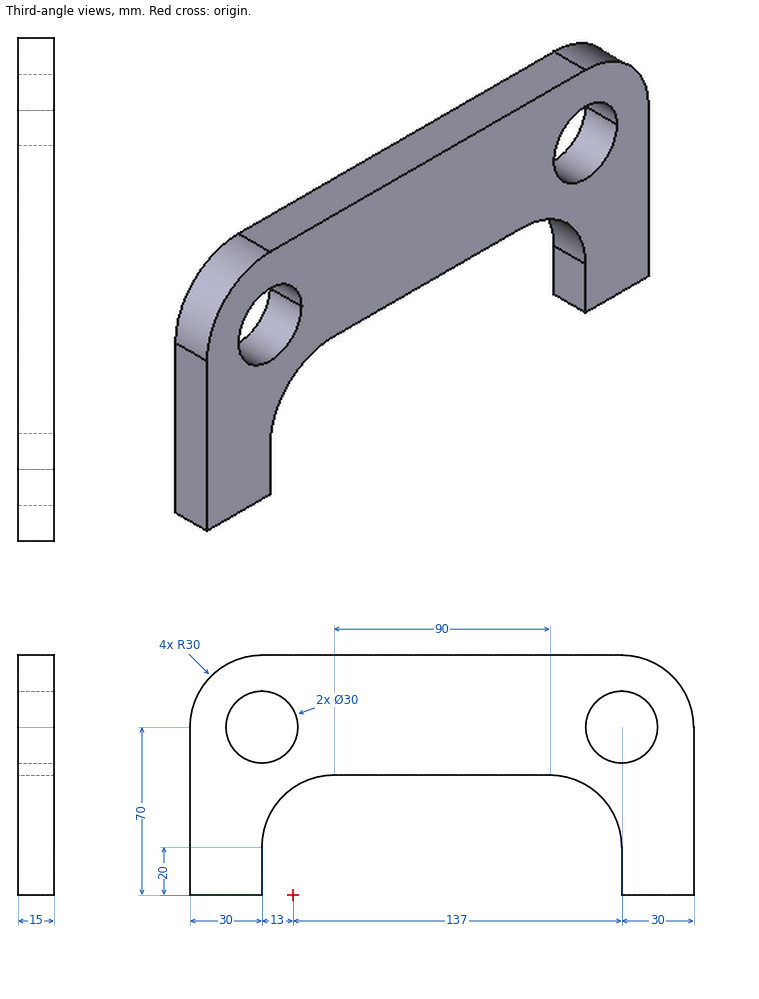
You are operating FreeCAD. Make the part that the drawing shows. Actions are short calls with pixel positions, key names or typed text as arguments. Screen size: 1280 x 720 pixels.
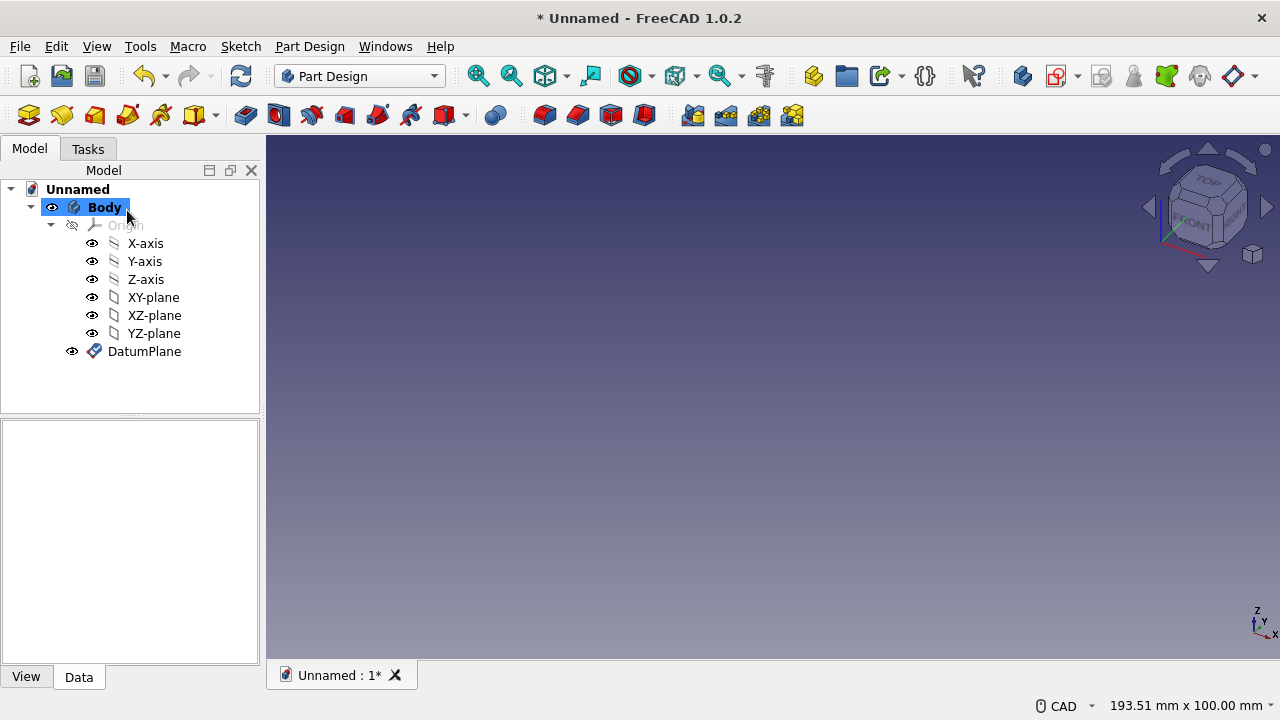
click(117, 351)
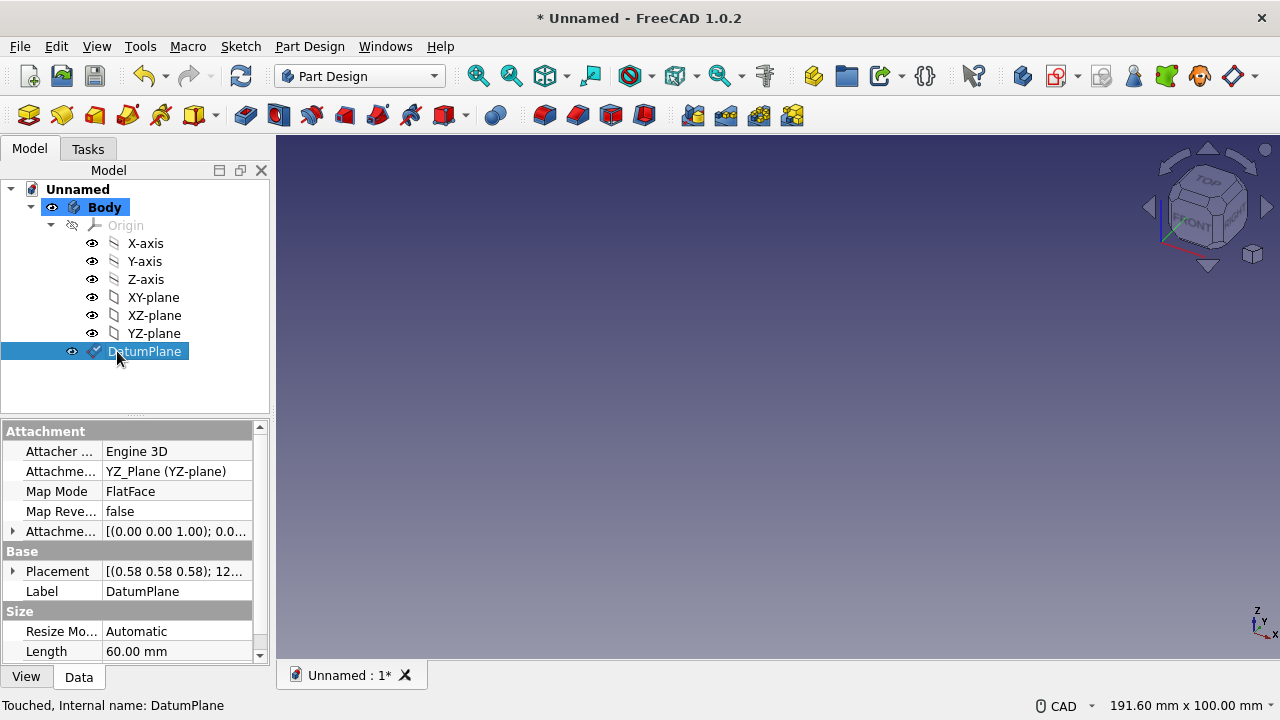
click(1056, 76)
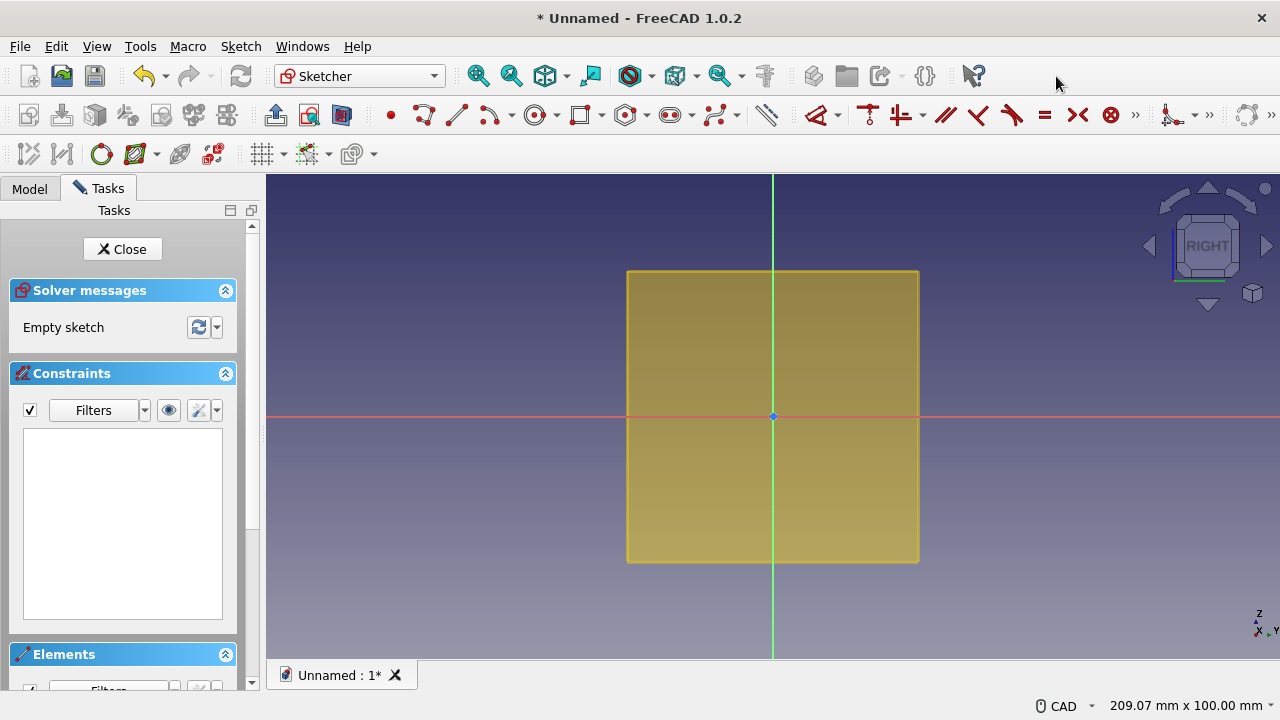
scroll(294, 631, down, 3)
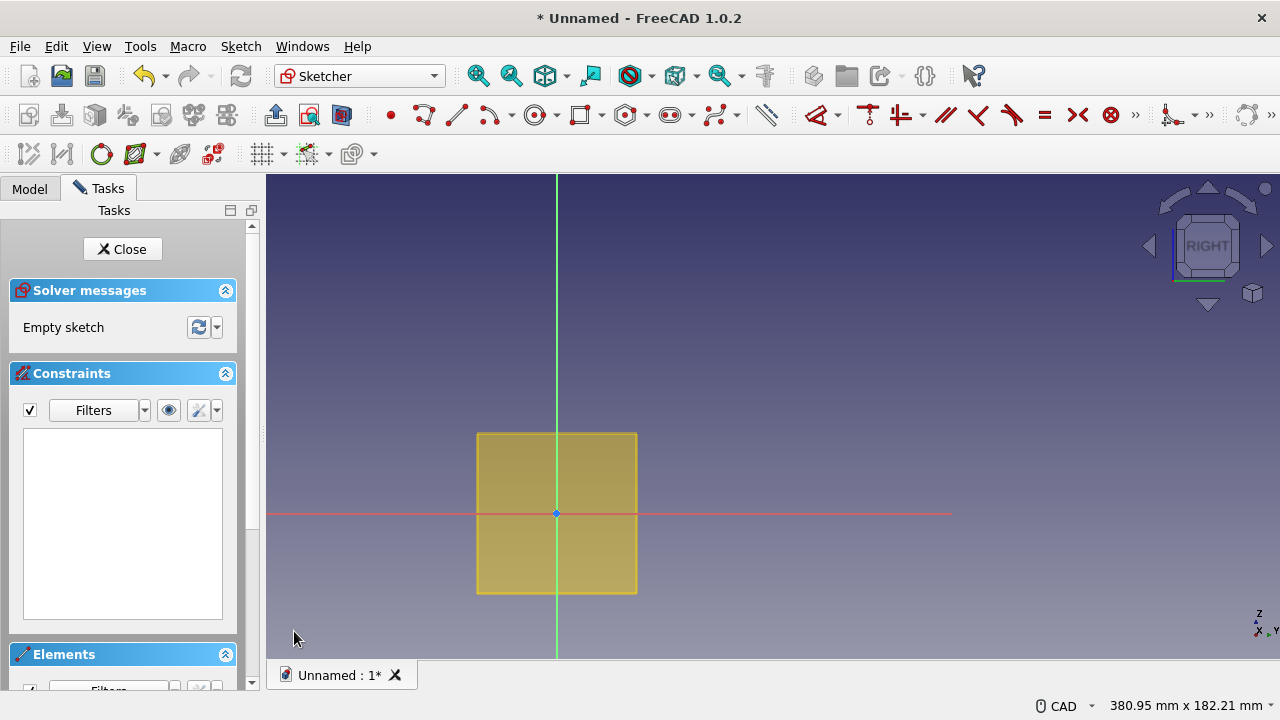
key(g)
key(m)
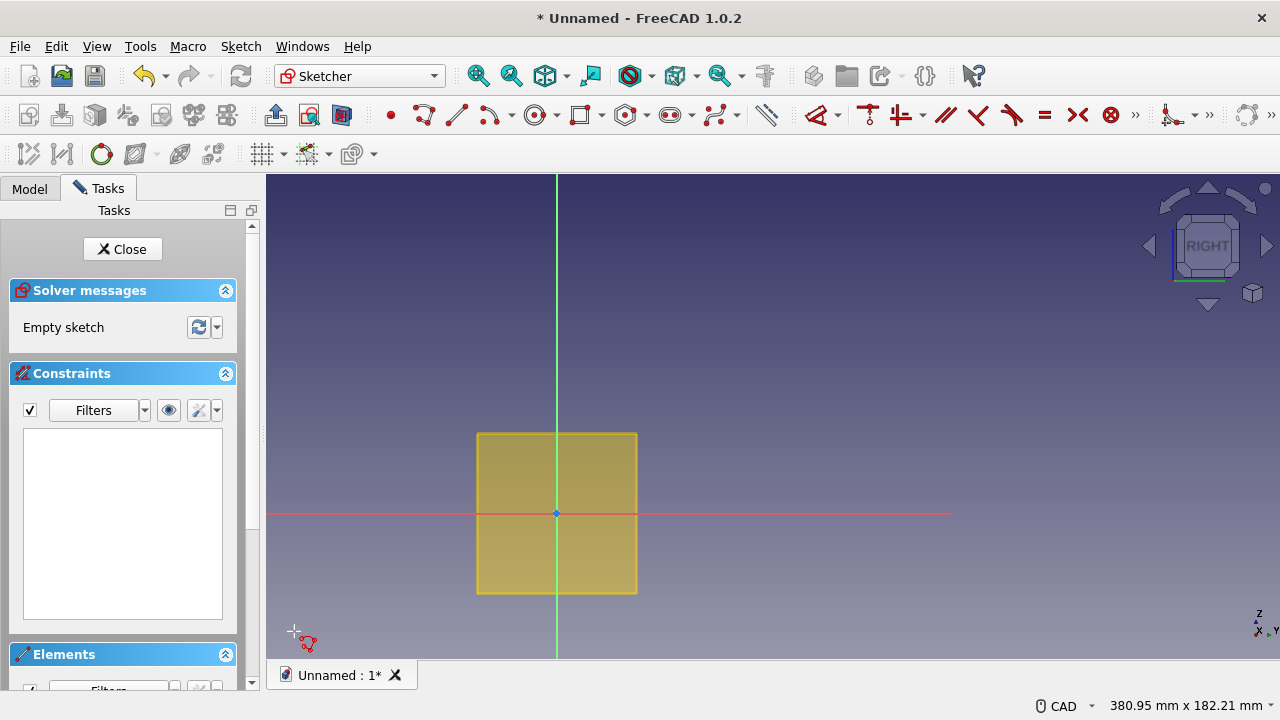
click(522, 460)
click(522, 514)
click(442, 505)
click(442, 327)
right_click(442, 327)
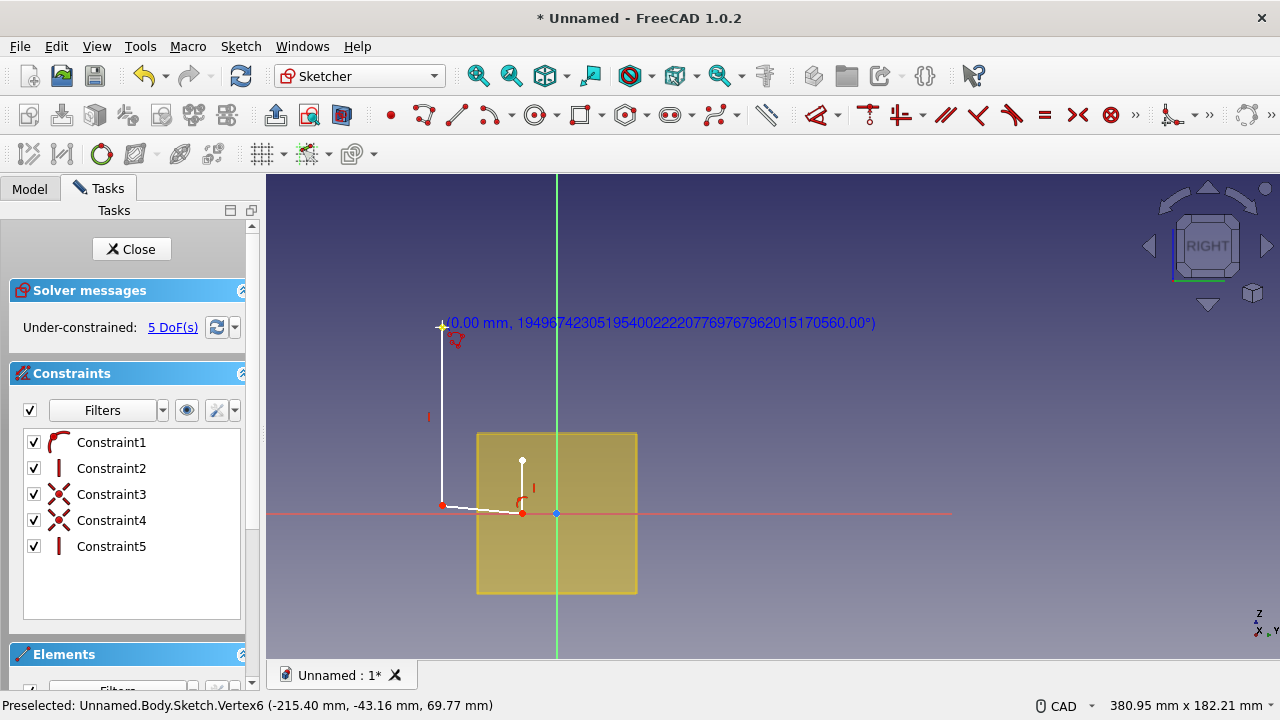
key(g)
key(l)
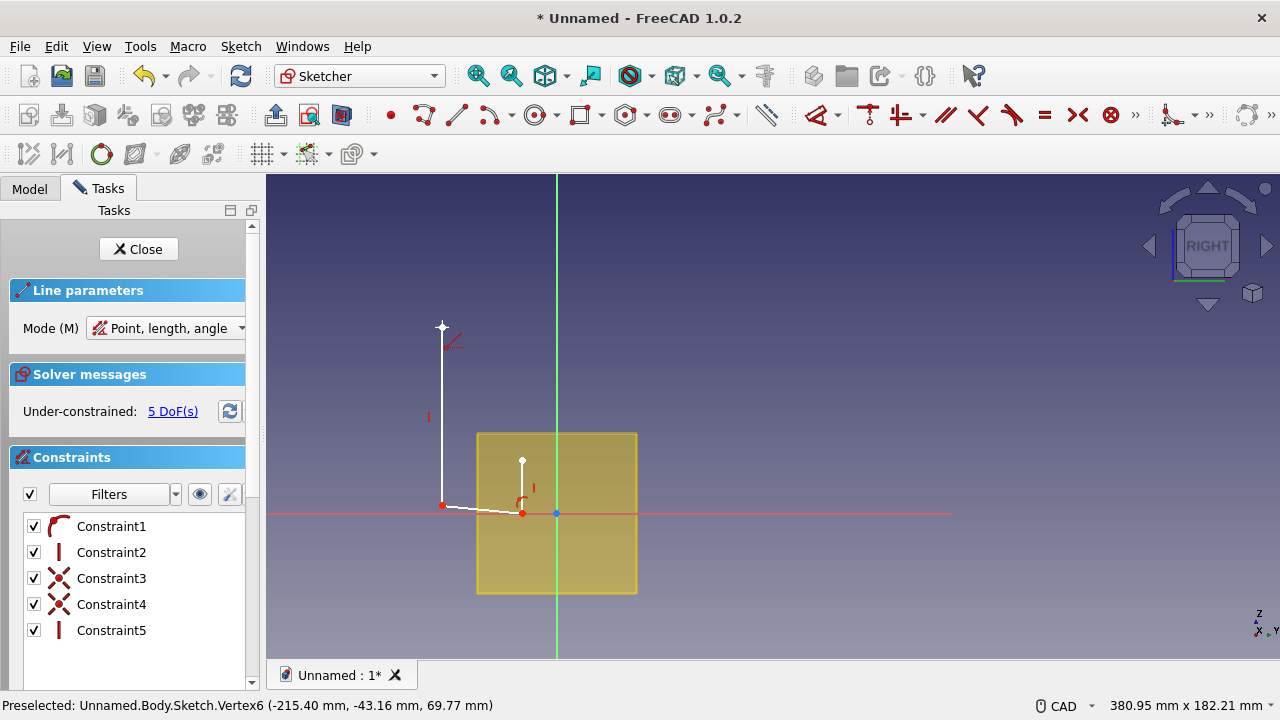
click(522, 248)
click(922, 248)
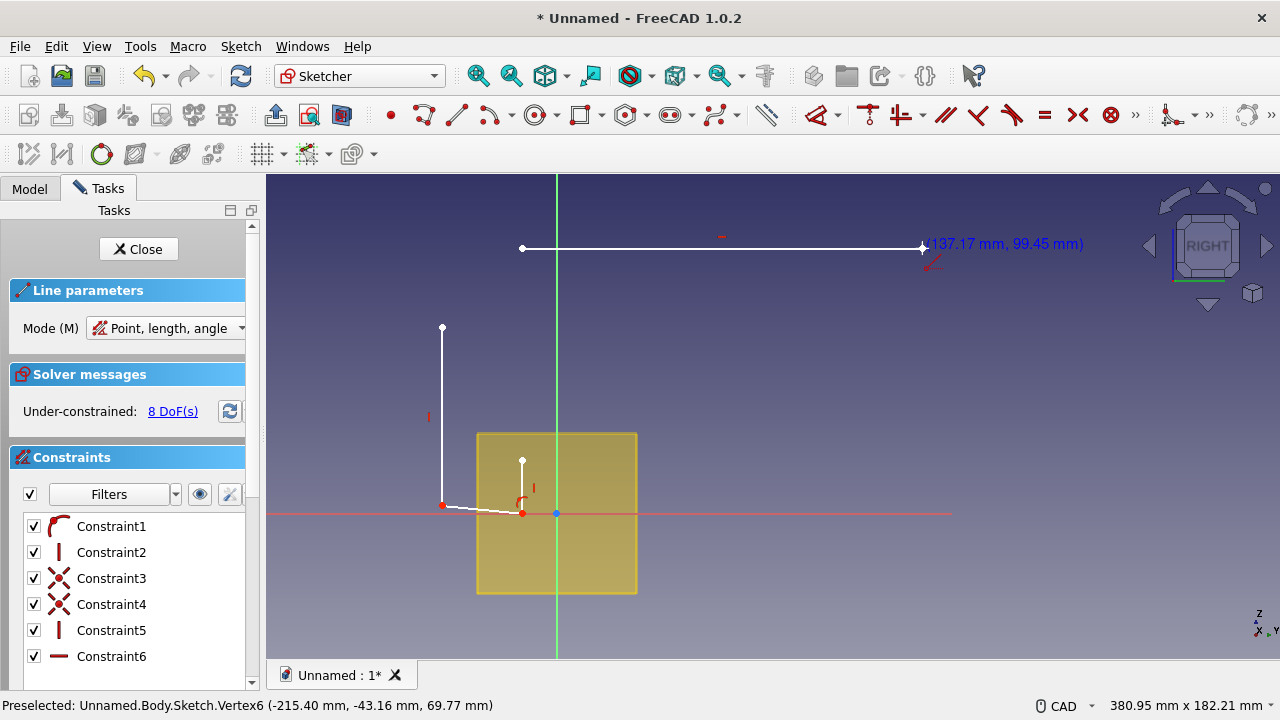
key(g)
key(m)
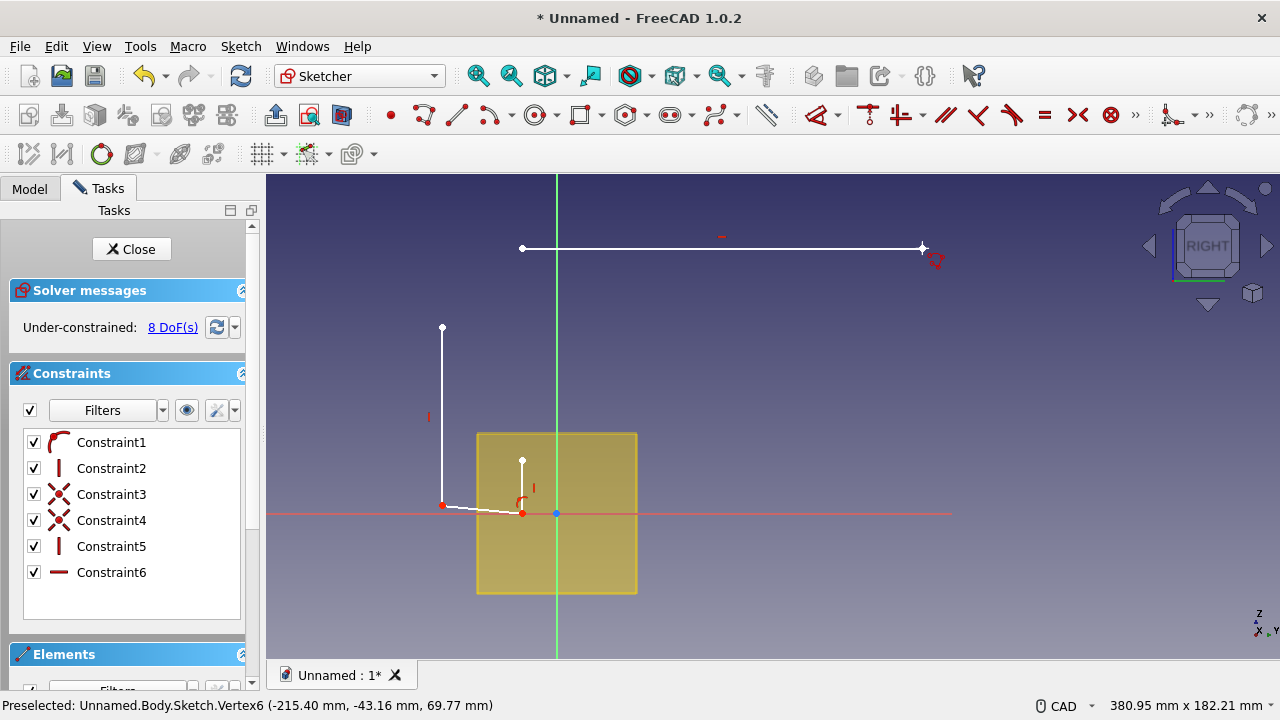
click(1001, 327)
click(1001, 514)
click(922, 505)
click(922, 460)
right_click(922, 460)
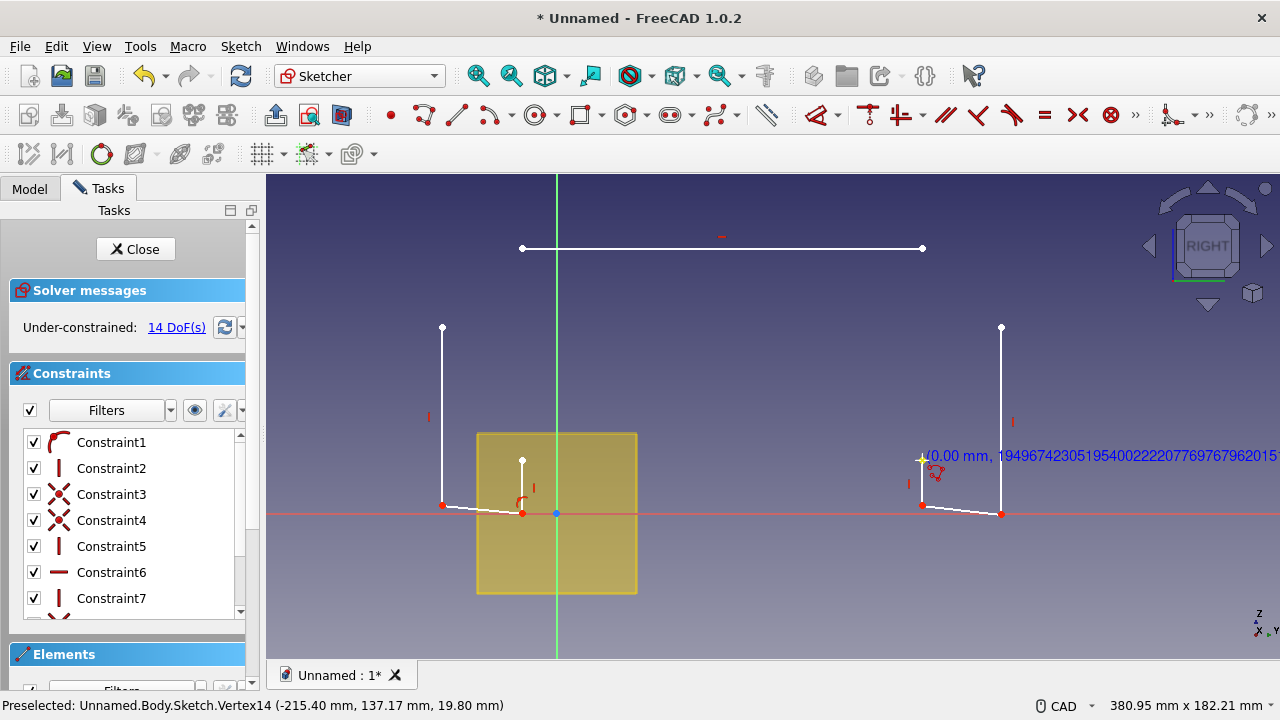
key(g)
key(l)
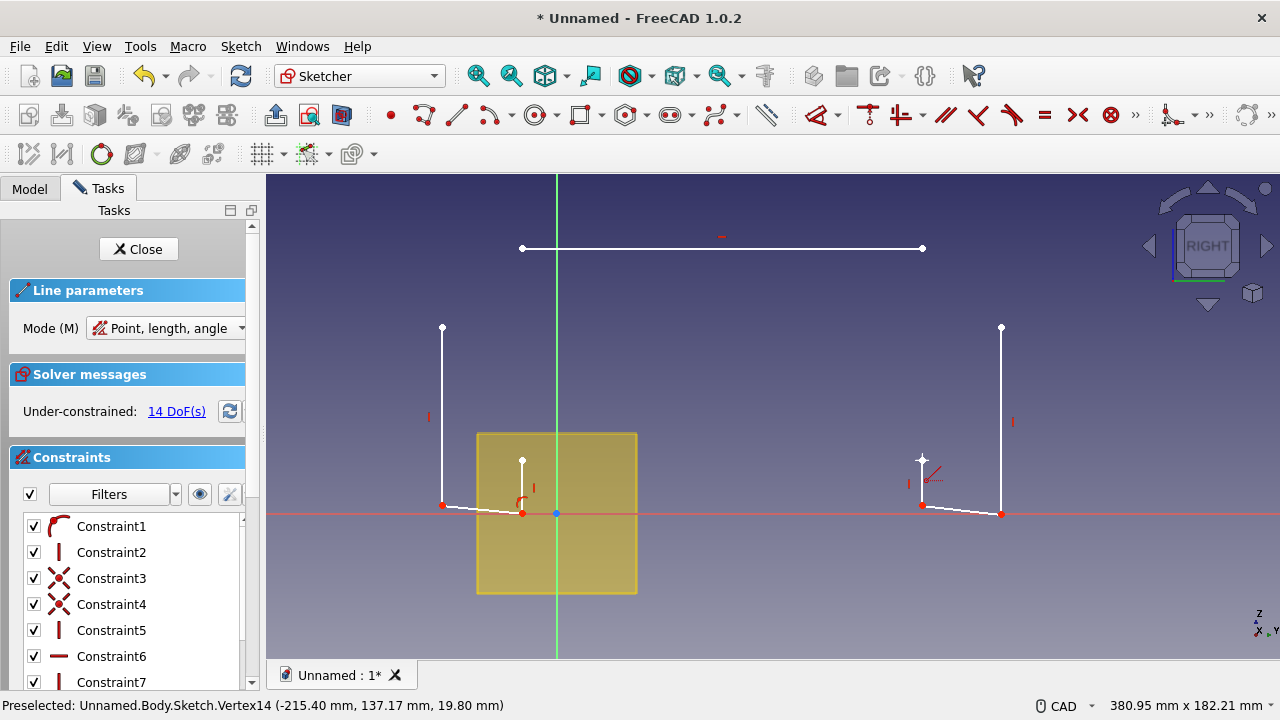
click(842, 381)
click(602, 381)